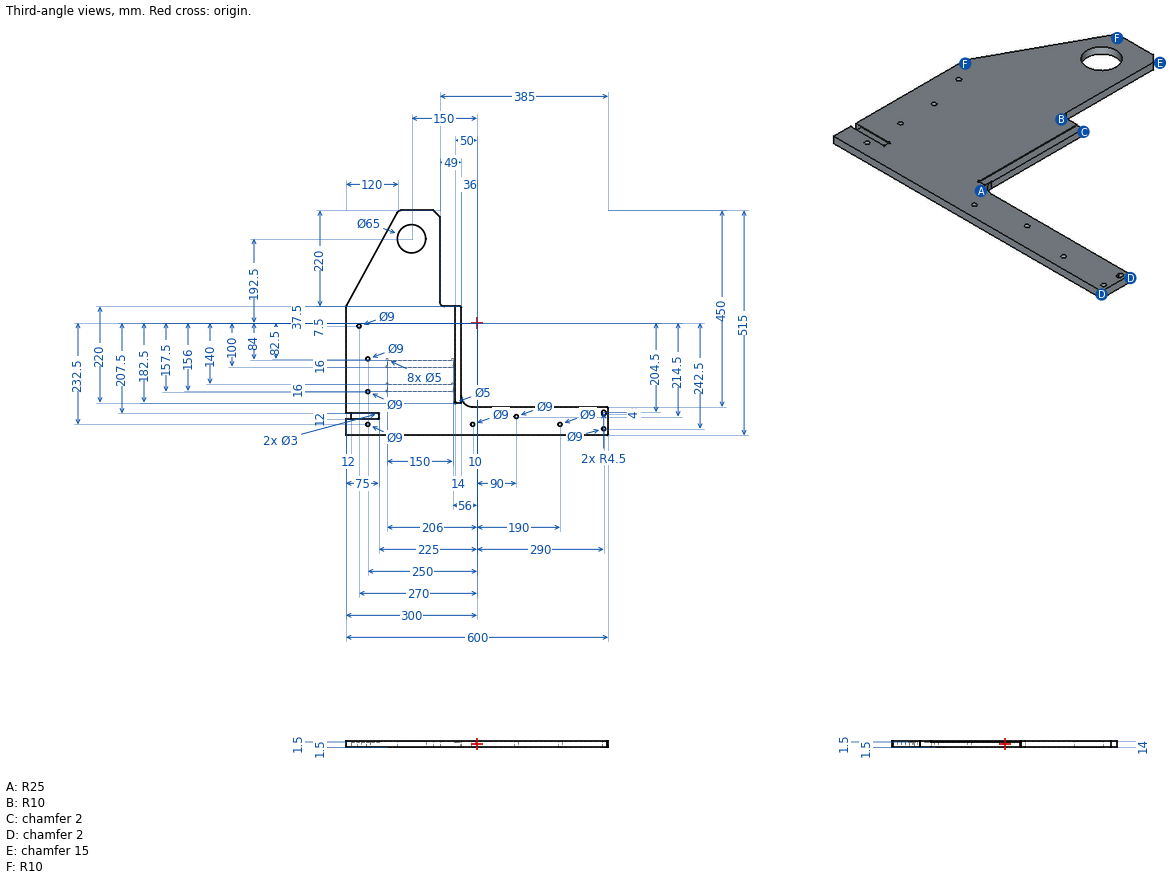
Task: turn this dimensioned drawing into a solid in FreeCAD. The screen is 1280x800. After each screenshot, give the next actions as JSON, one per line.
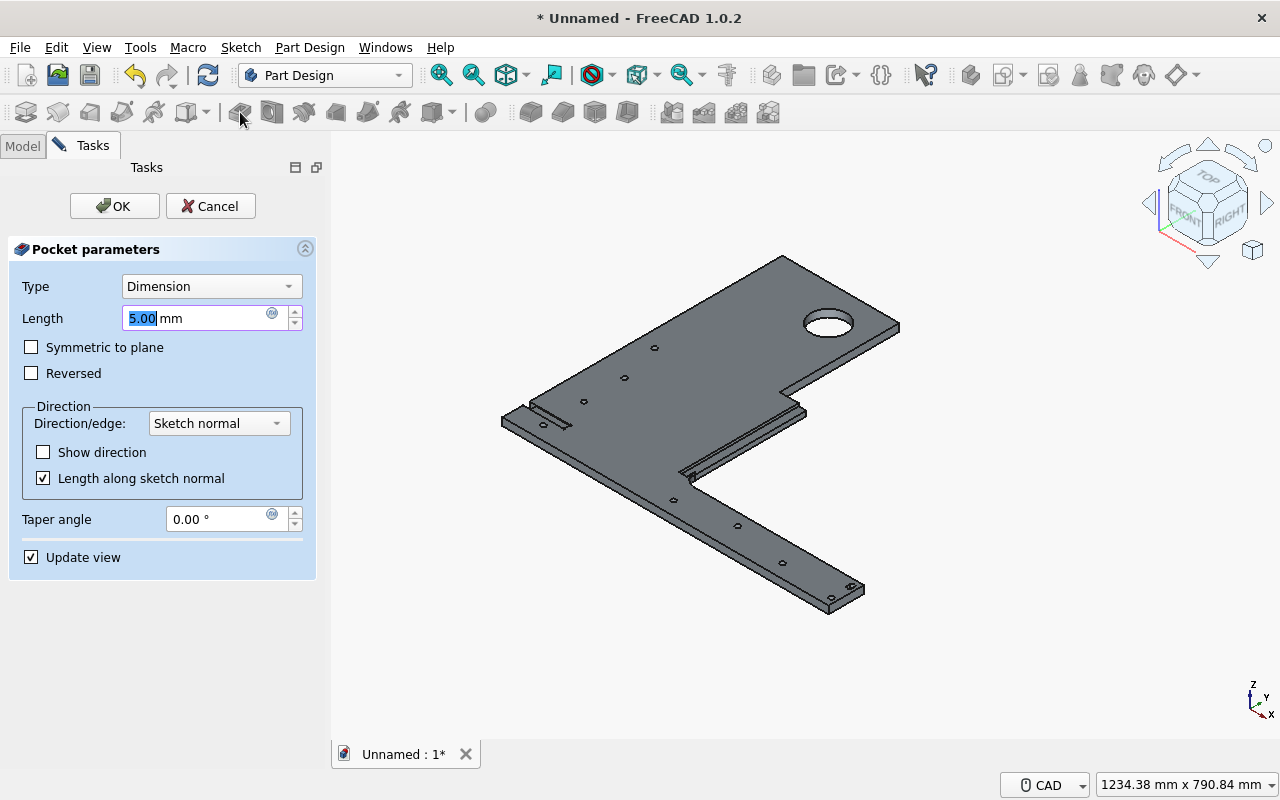
{"action": "type", "text": "1.5"}
{"action": "key", "text": "Tab"}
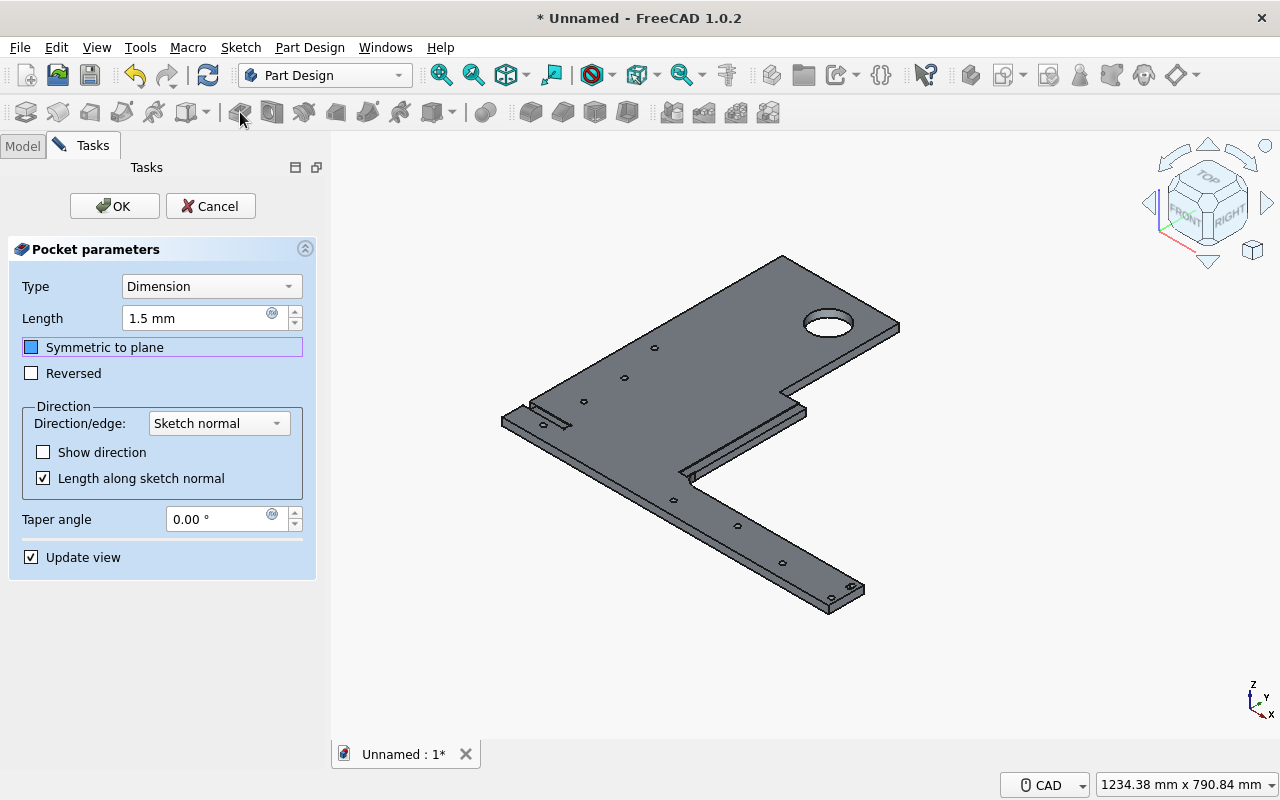
{"action": "left_click", "coordinate": [115, 206]}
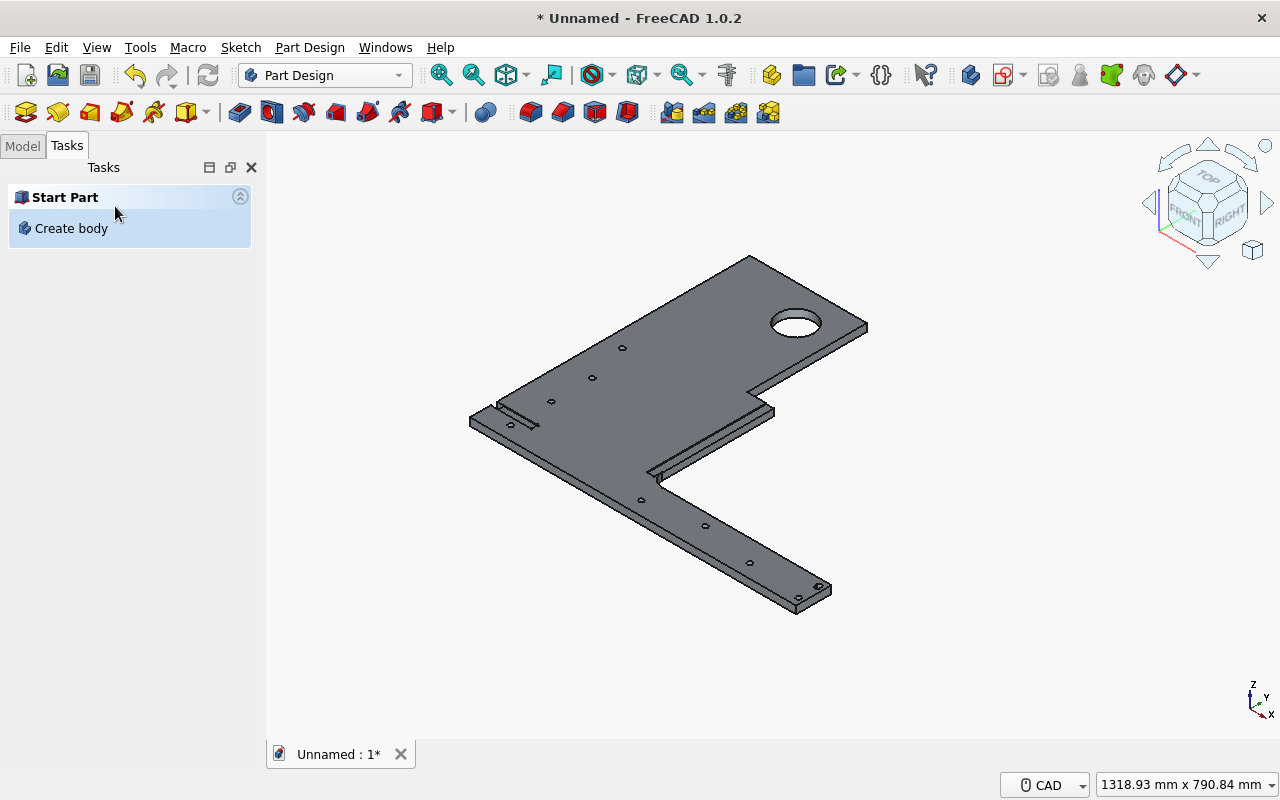
{"action": "left_click", "coordinate": [680, 376]}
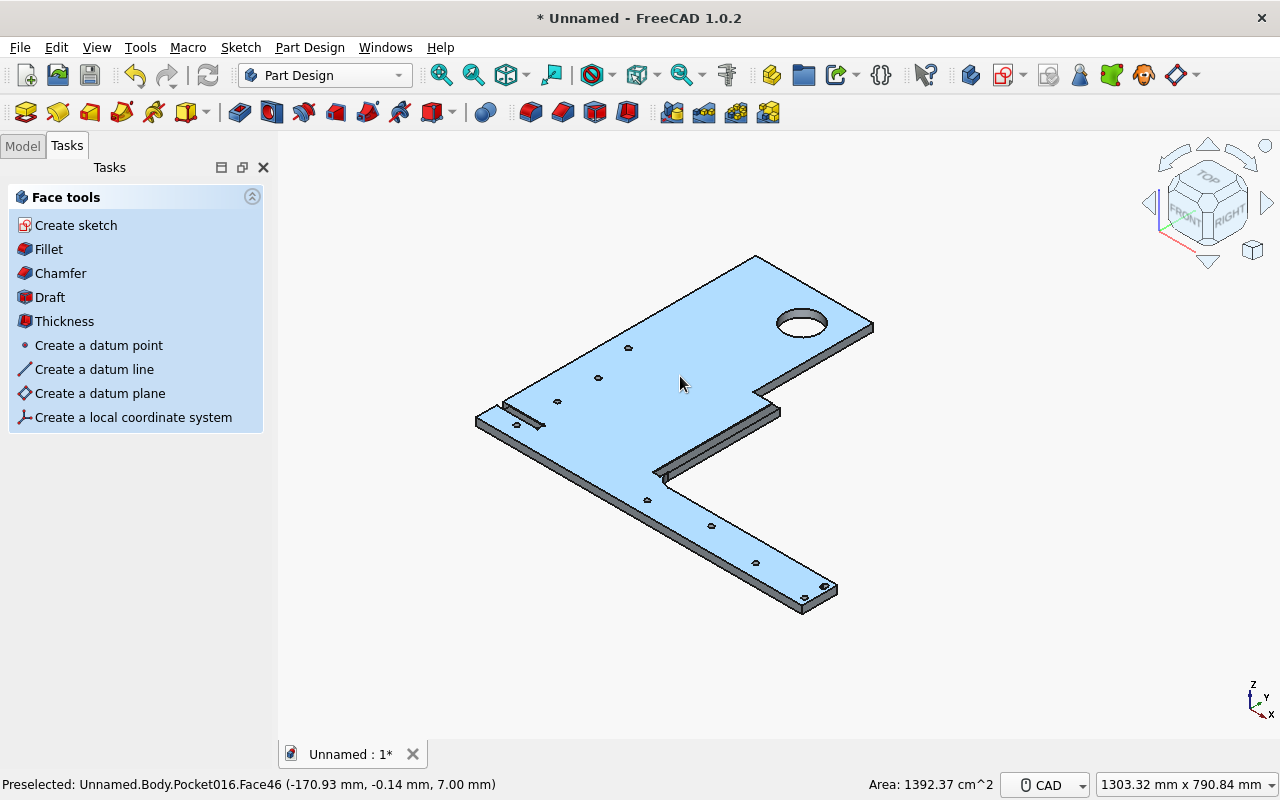
{"action": "left_click", "coordinate": [1004, 76]}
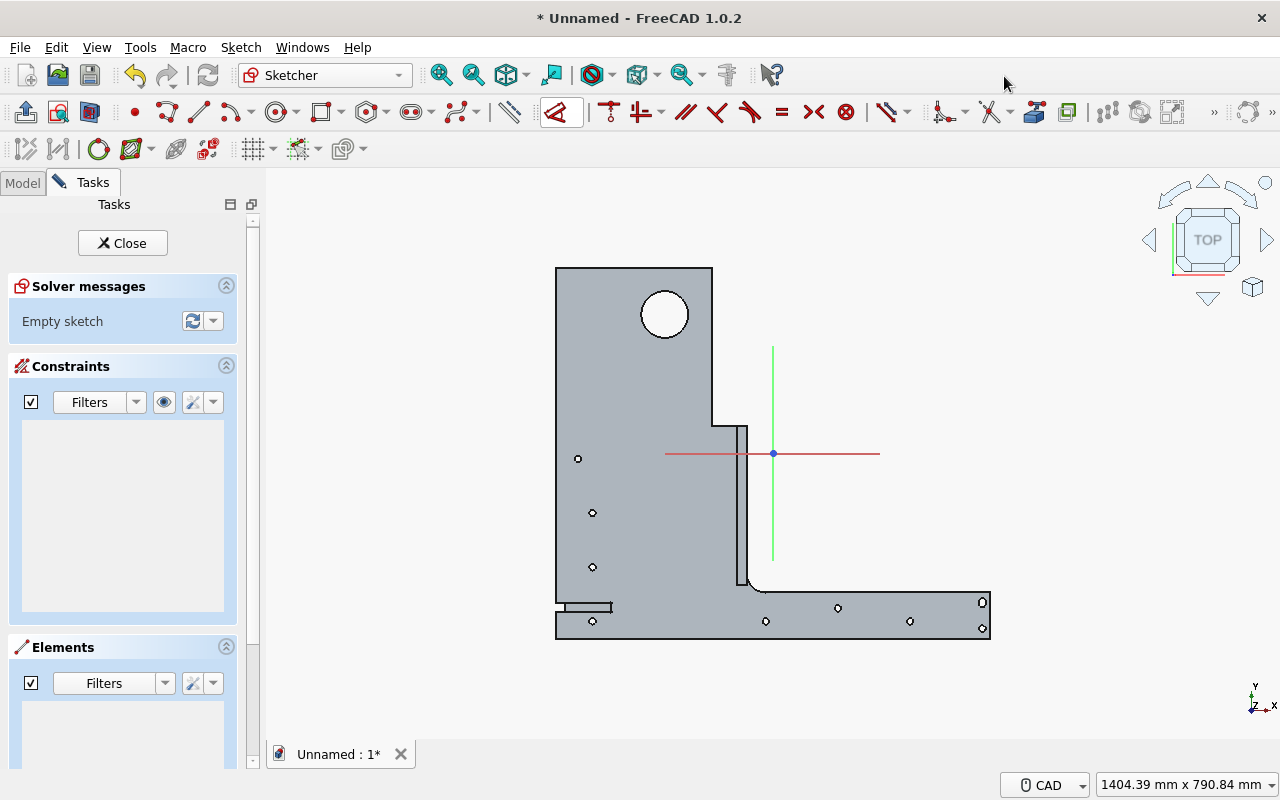
{"action": "scroll", "coordinate": [739, 592], "scroll_direction": "up", "scroll_amount": 15}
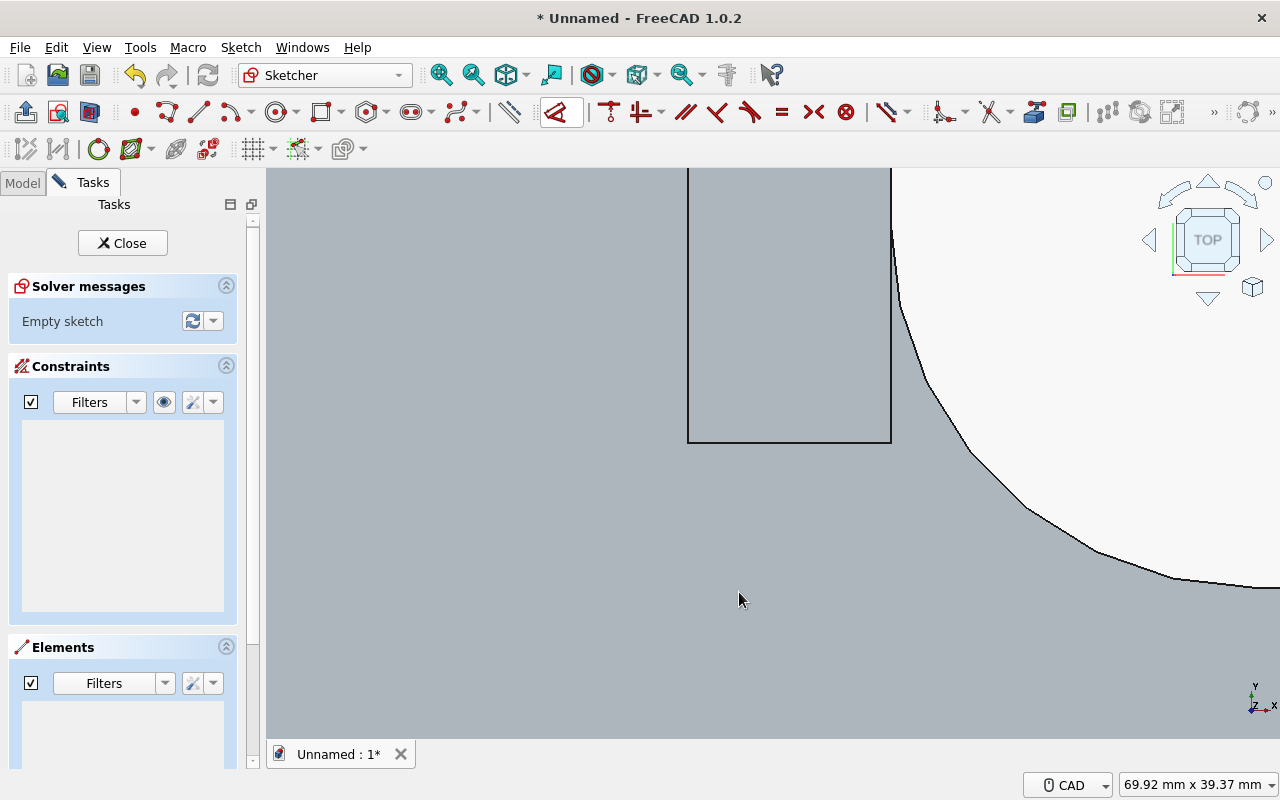
{"action": "scroll", "coordinate": [684, 440], "scroll_direction": "up", "scroll_amount": 8}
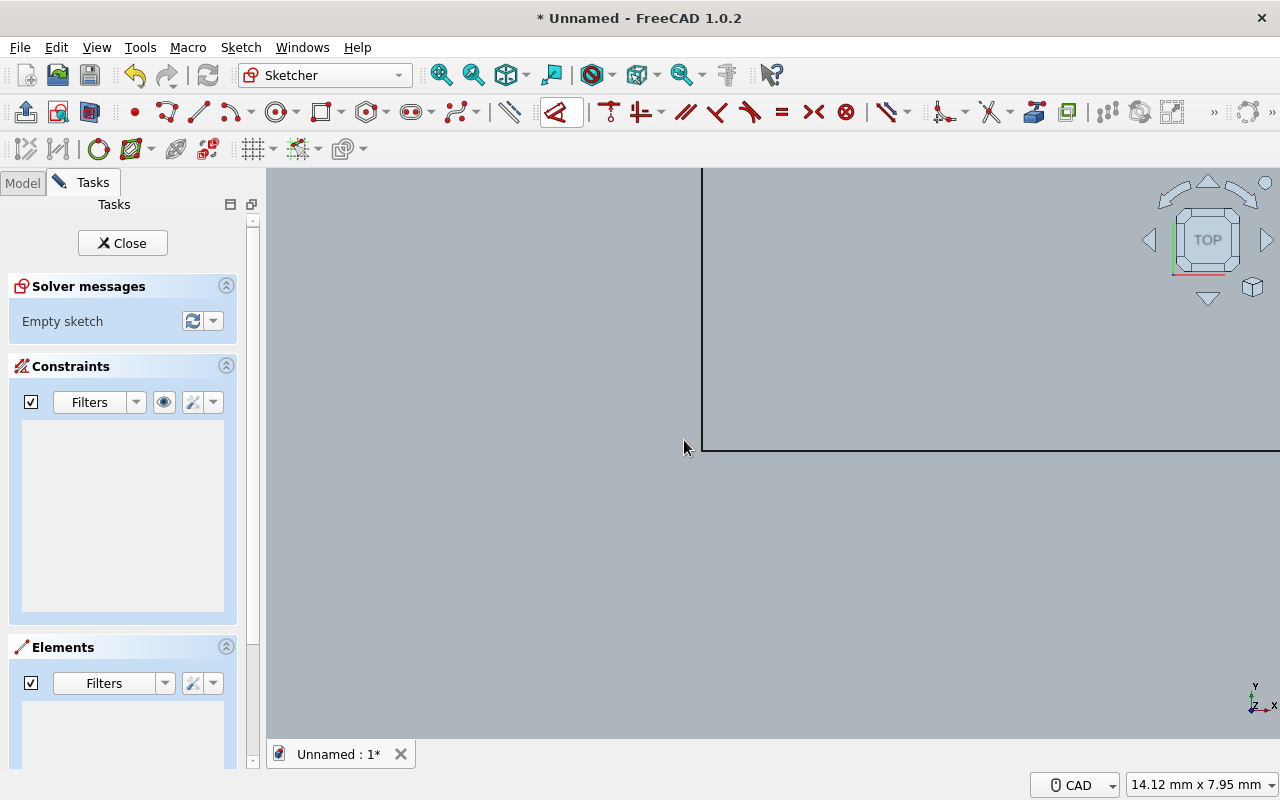
{"action": "left_click", "coordinate": [276, 112]}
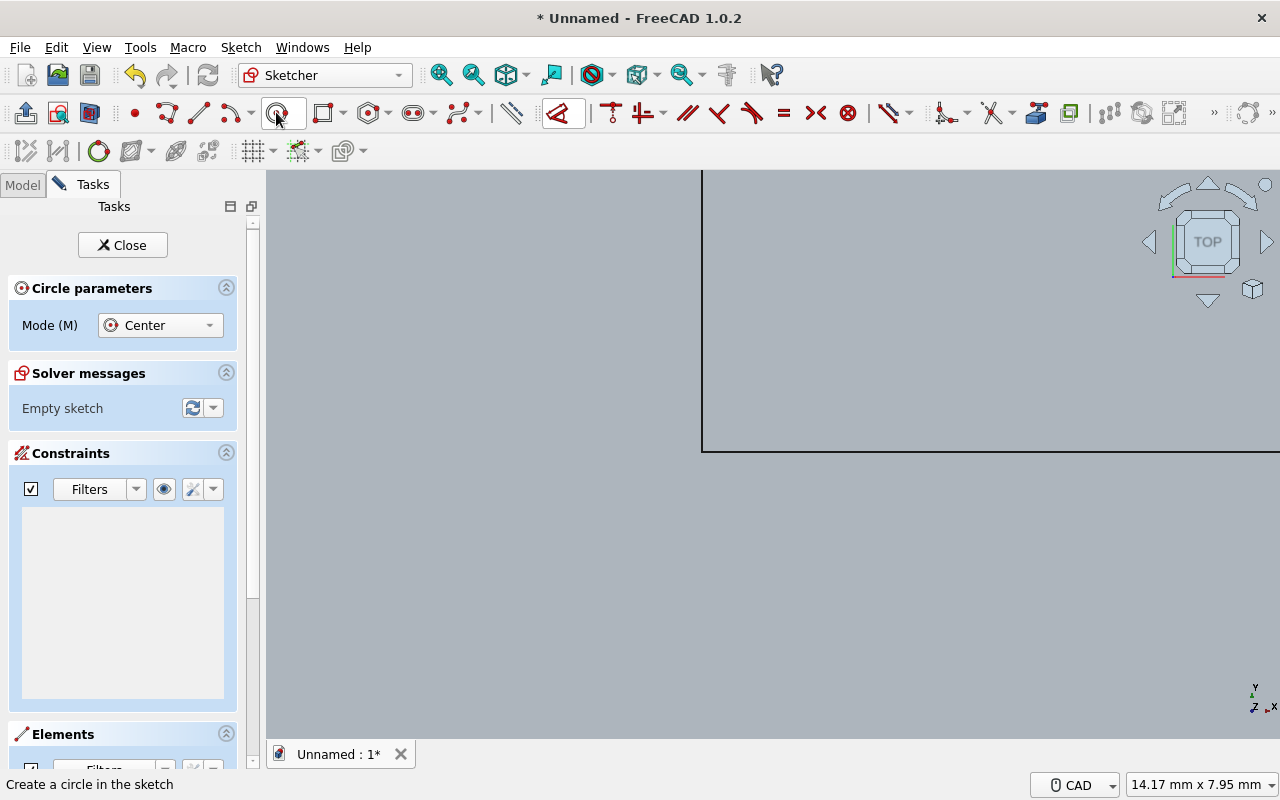
{"action": "left_click", "coordinate": [702, 452]}
{"action": "mouse_move", "coordinate": [828, 325]}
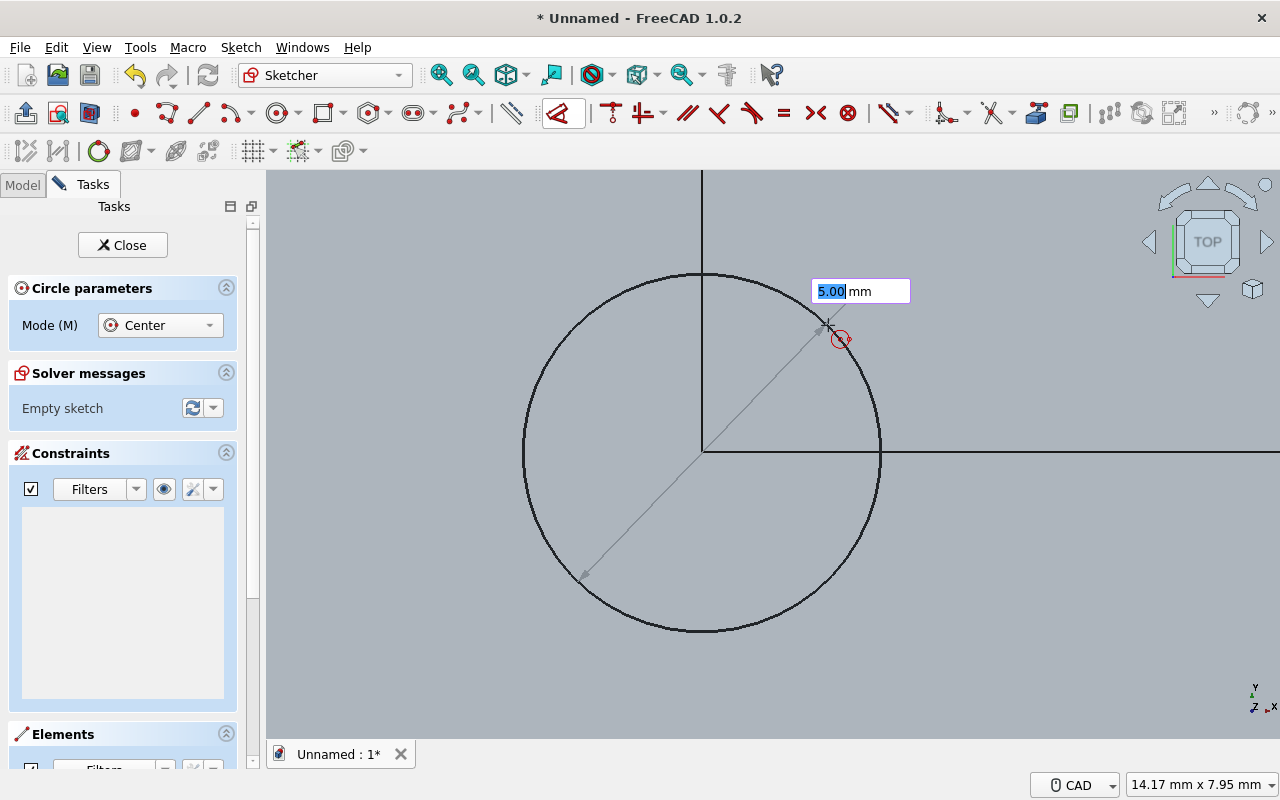
{"action": "type", "text": "5"}
{"action": "key", "text": "Return"}
{"action": "key", "text": "Escape"}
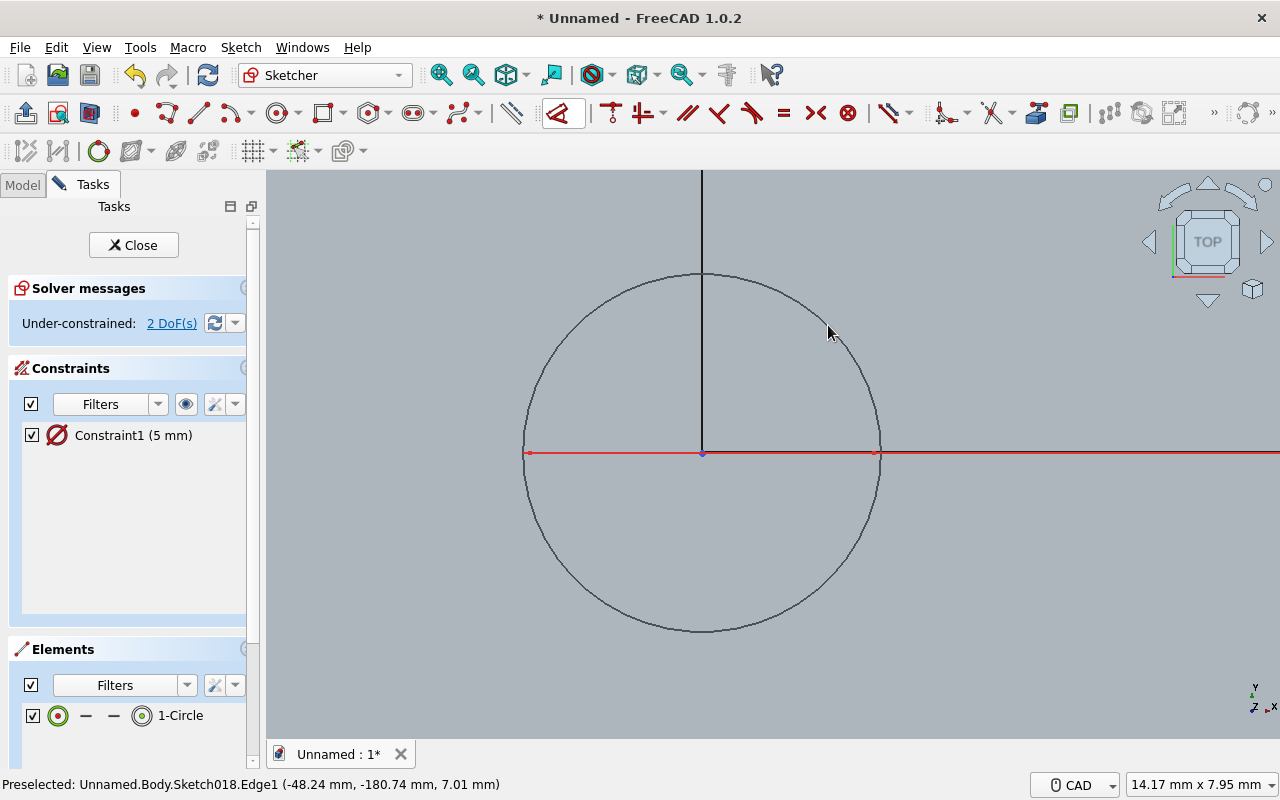
{"action": "left_click", "coordinate": [702, 453]}